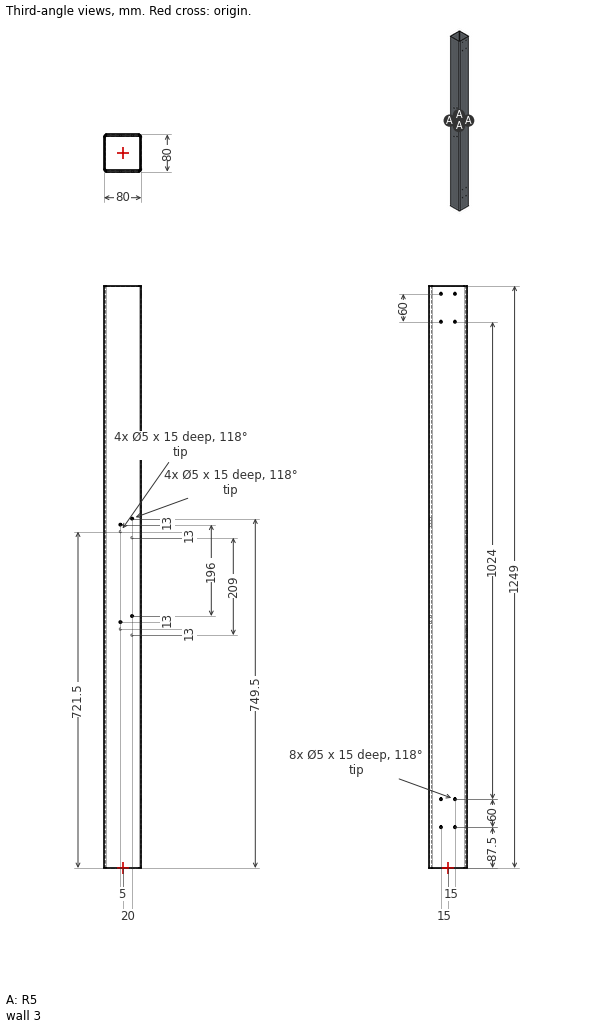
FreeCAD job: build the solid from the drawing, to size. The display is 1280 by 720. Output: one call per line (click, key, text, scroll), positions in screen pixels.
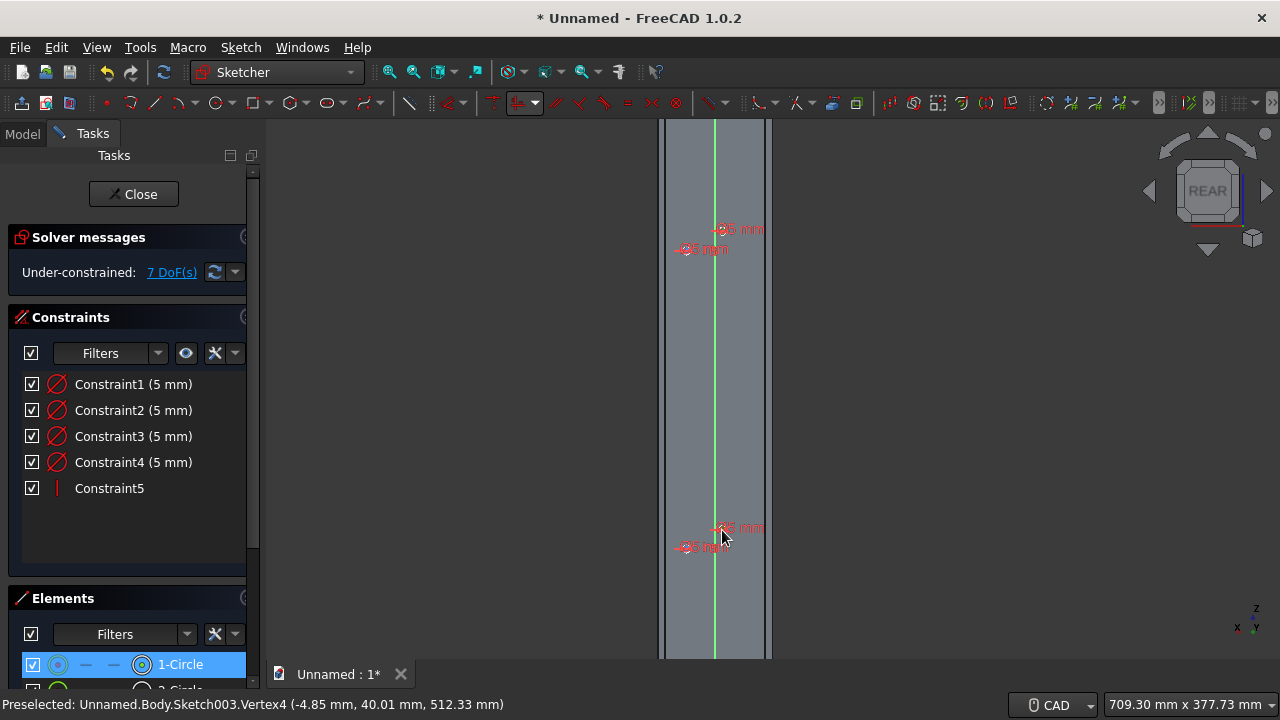
key(v)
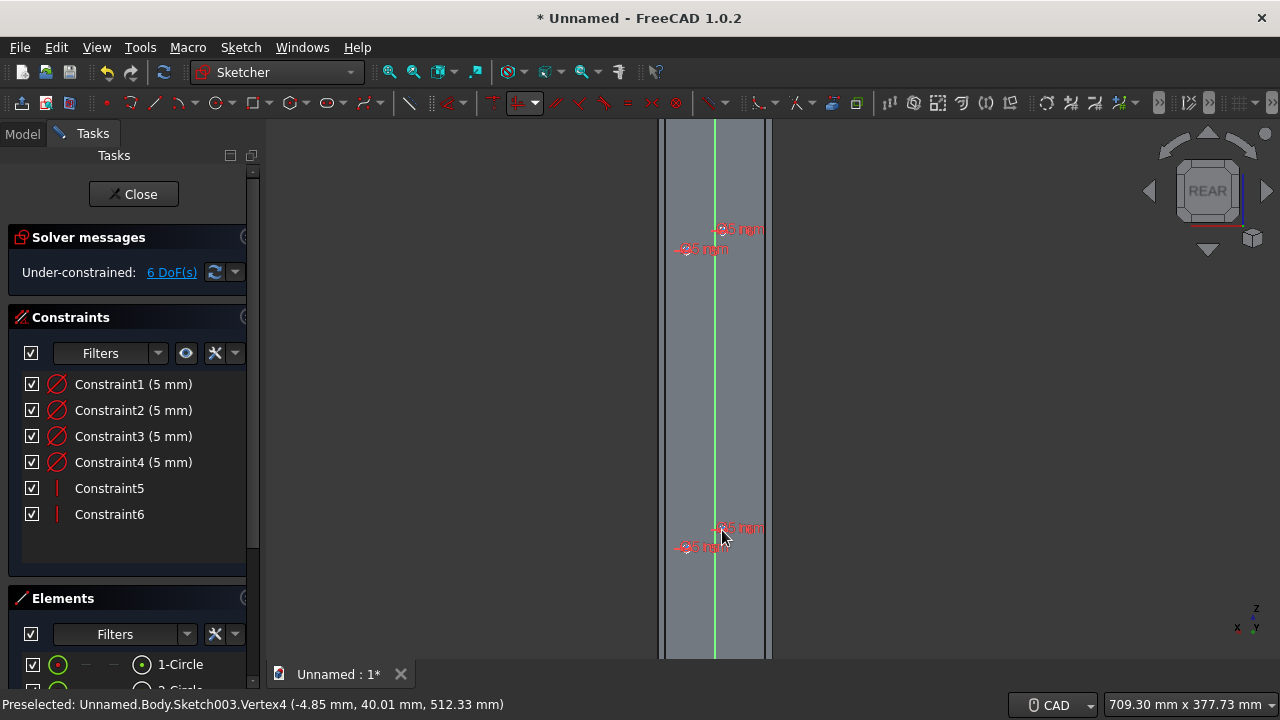
key(d)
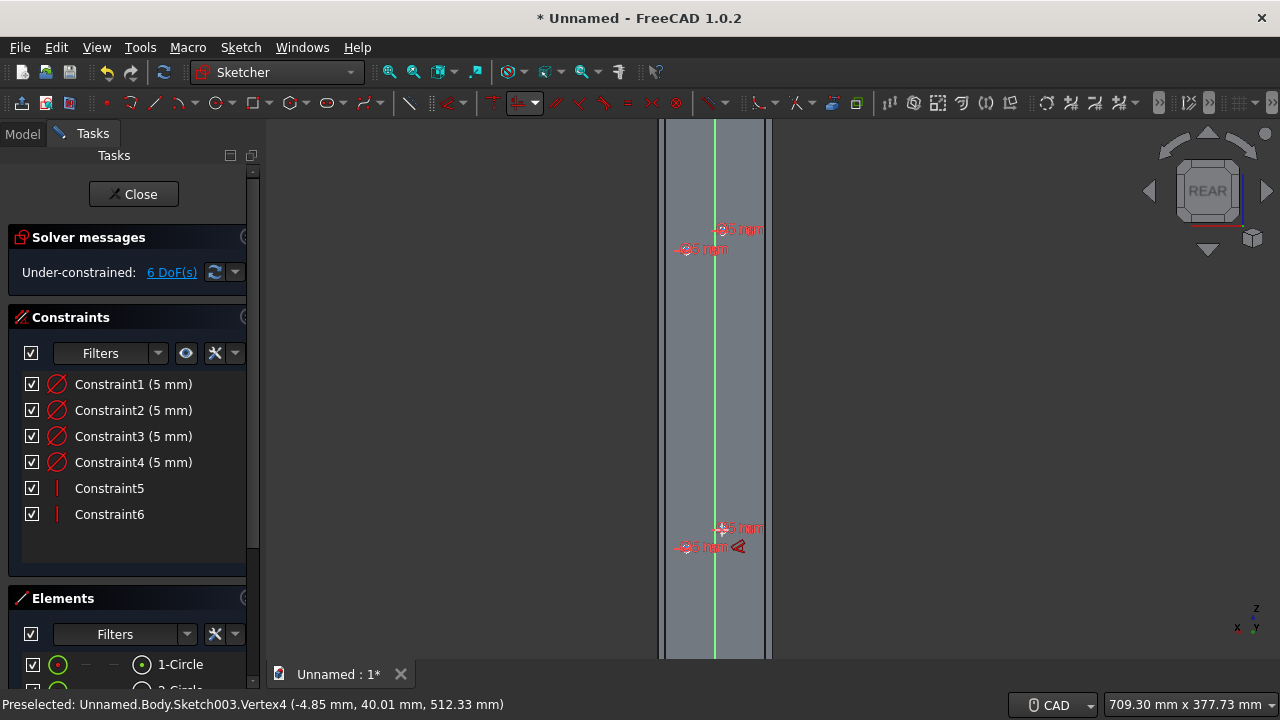
scroll(723, 231, up, 9)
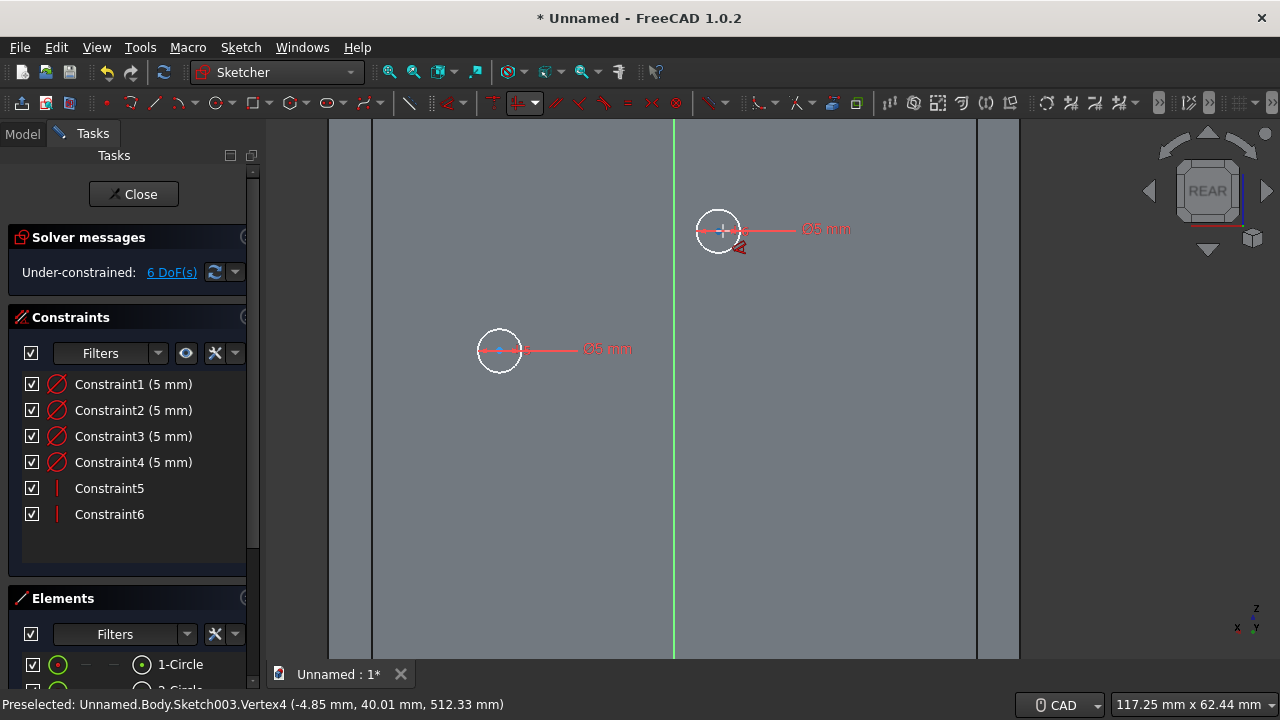
click(718, 231)
click(696, 197)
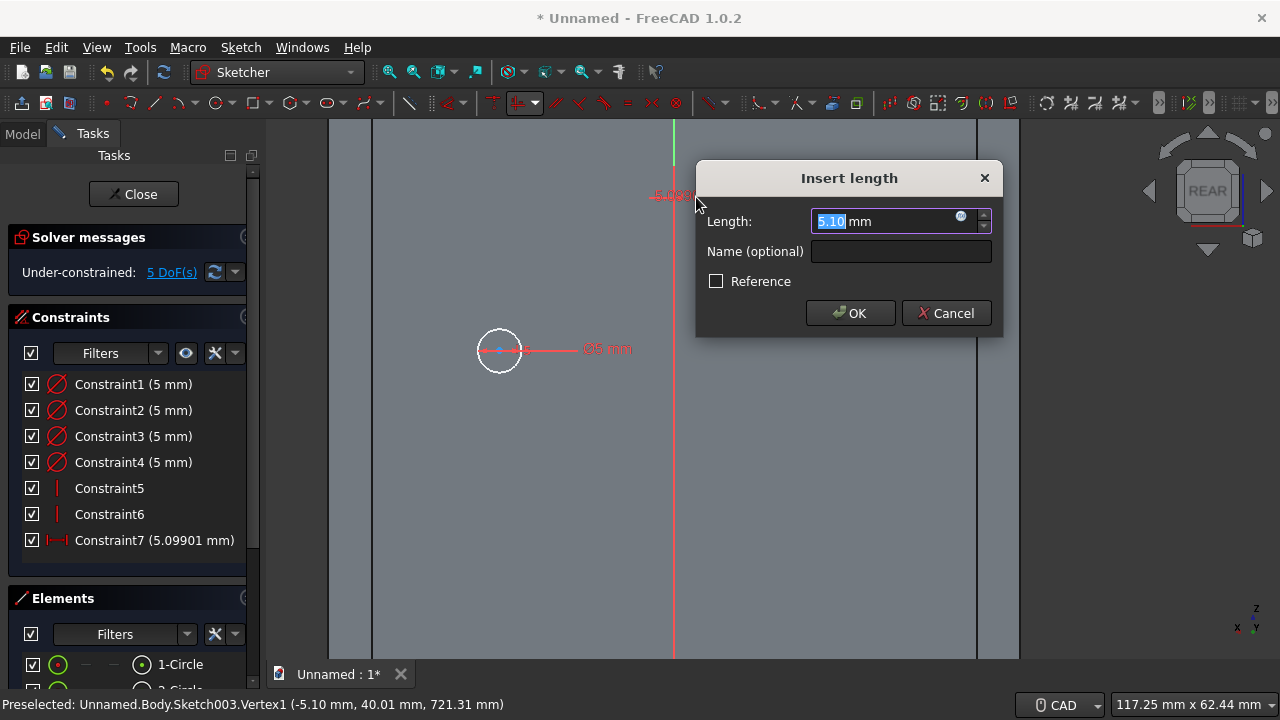
text(5)
key(Return)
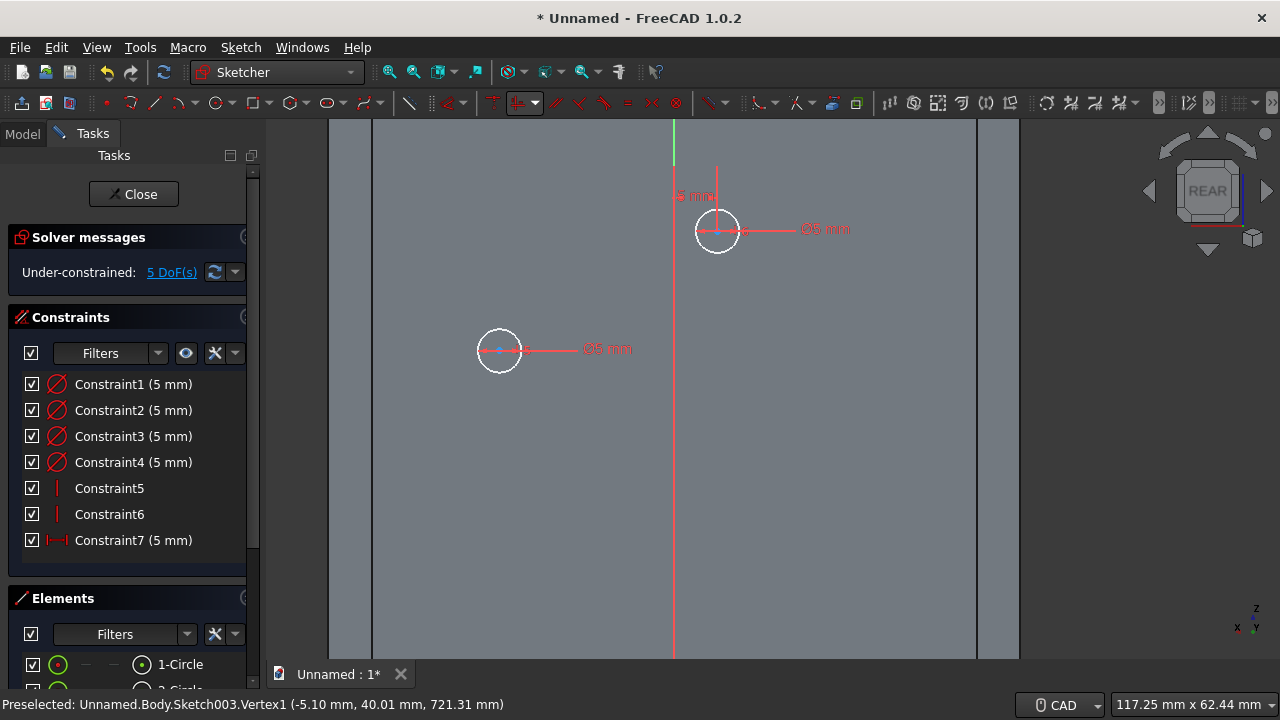
scroll(723, 230, down, 9)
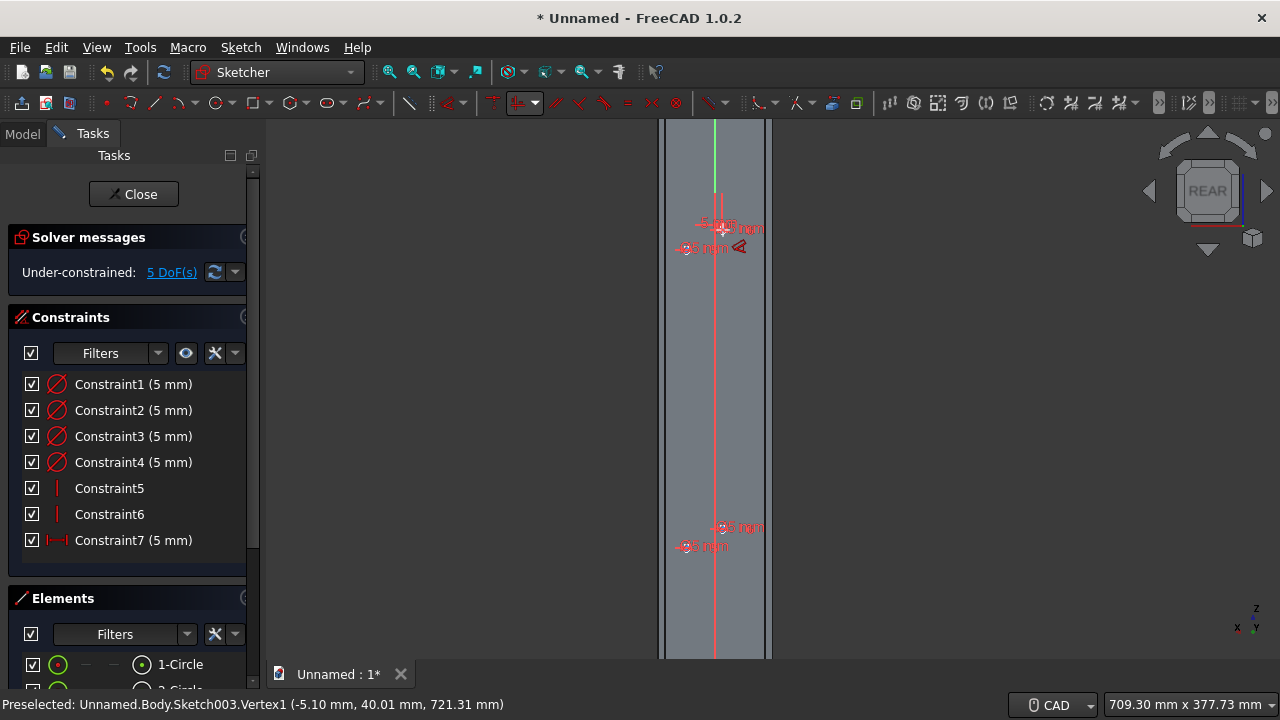
scroll(686, 250, up, 2)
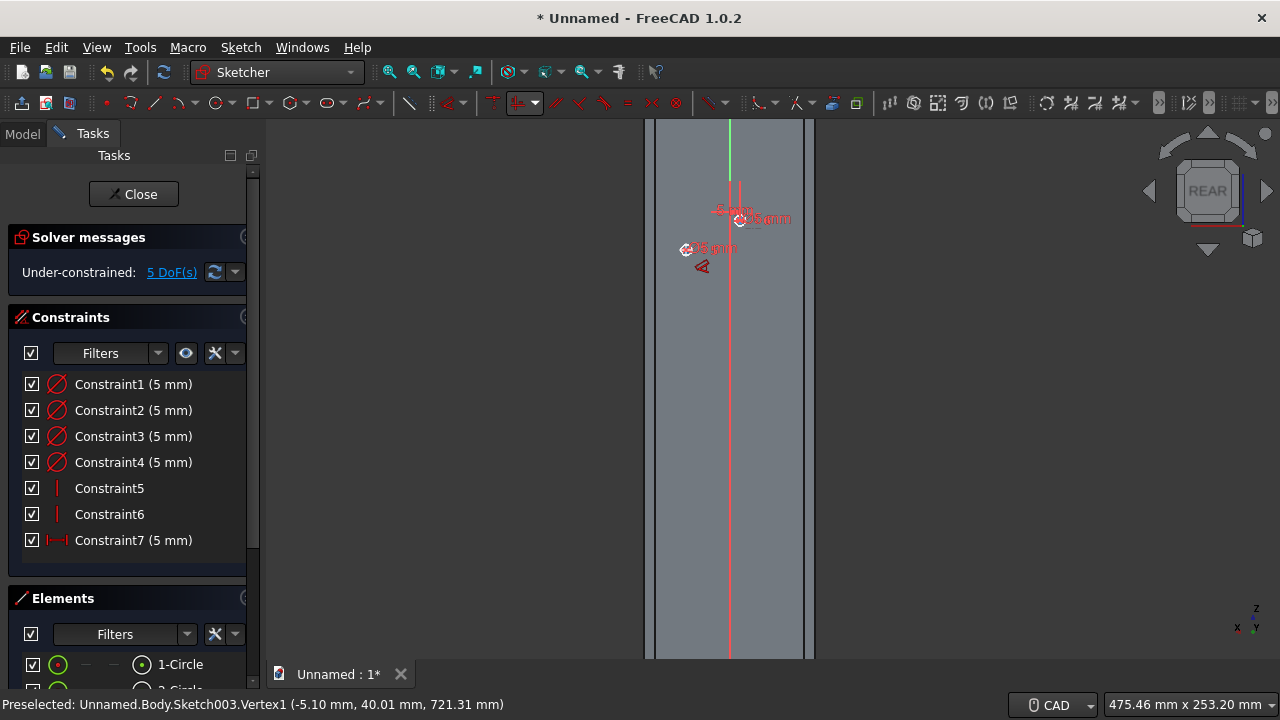
click(686, 250)
click(708, 192)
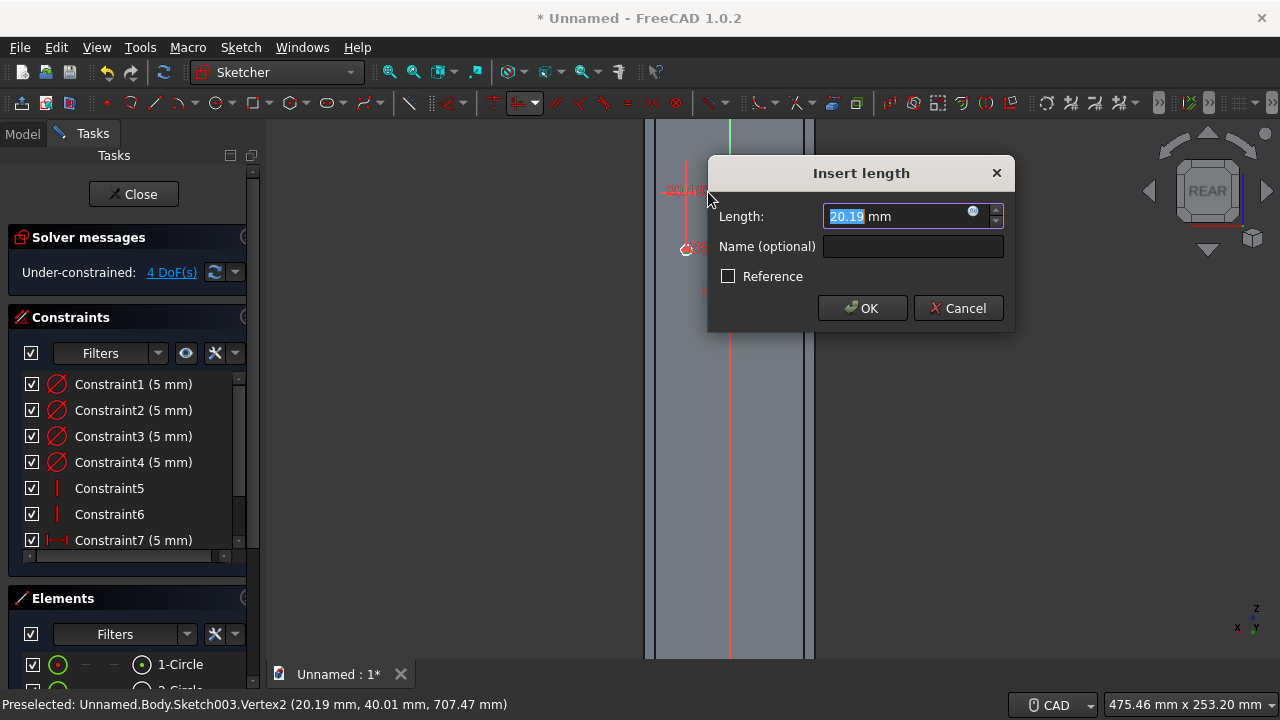
text(20)
key(Return)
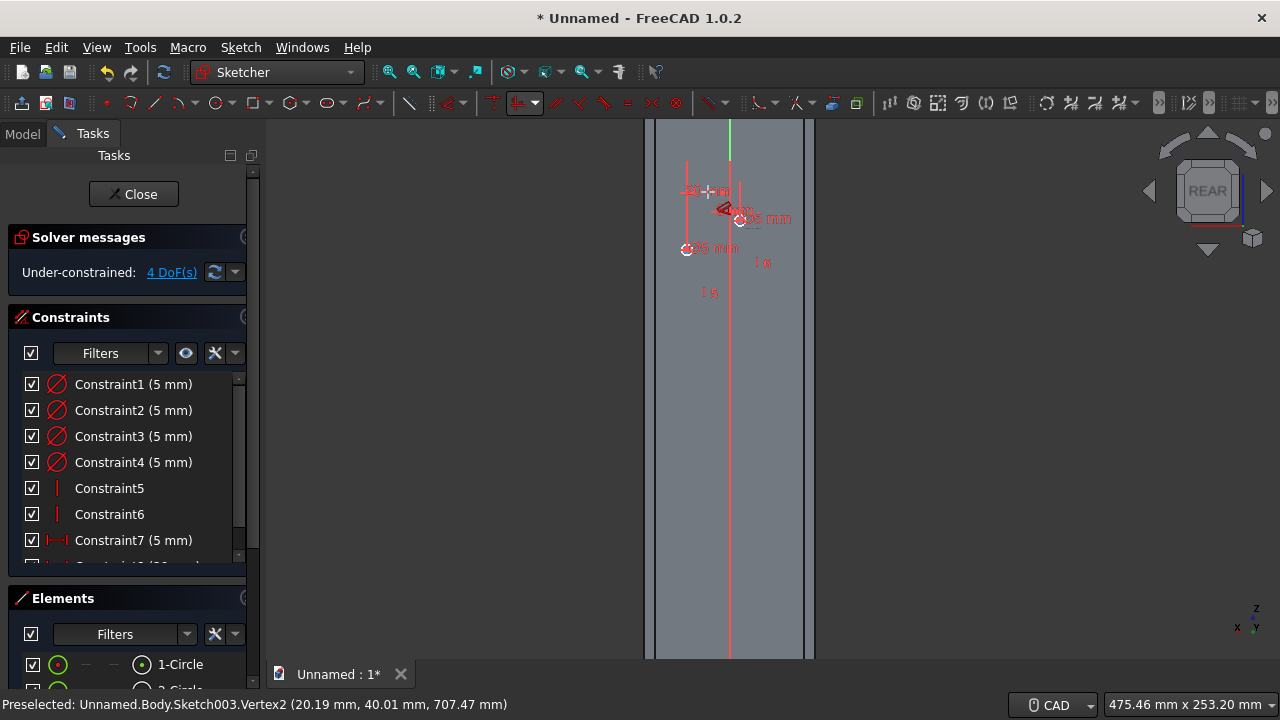
scroll(740, 221, up, 2)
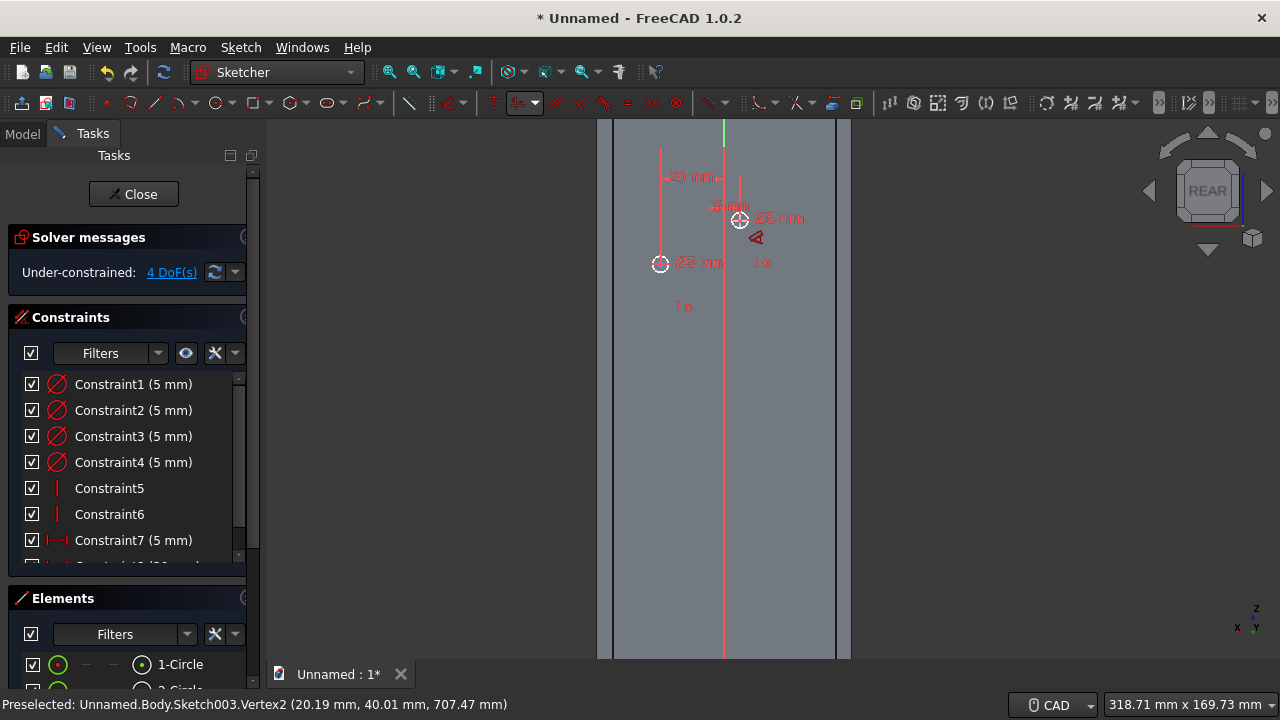
click(740, 220)